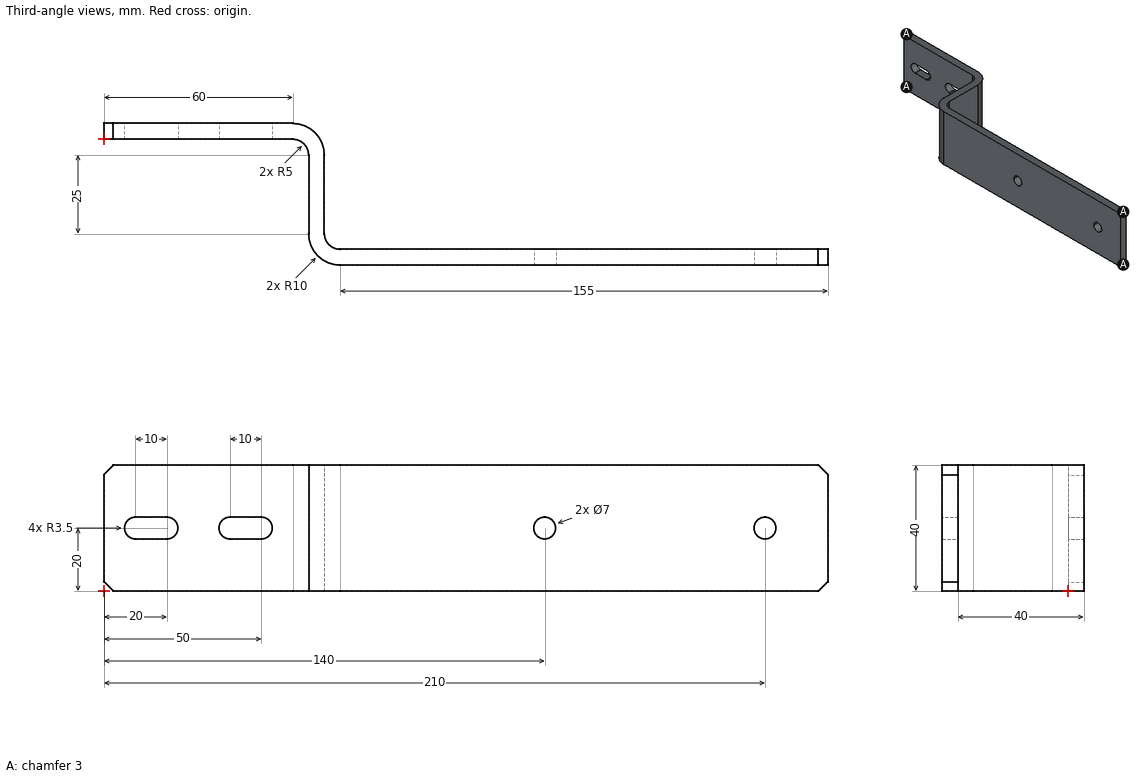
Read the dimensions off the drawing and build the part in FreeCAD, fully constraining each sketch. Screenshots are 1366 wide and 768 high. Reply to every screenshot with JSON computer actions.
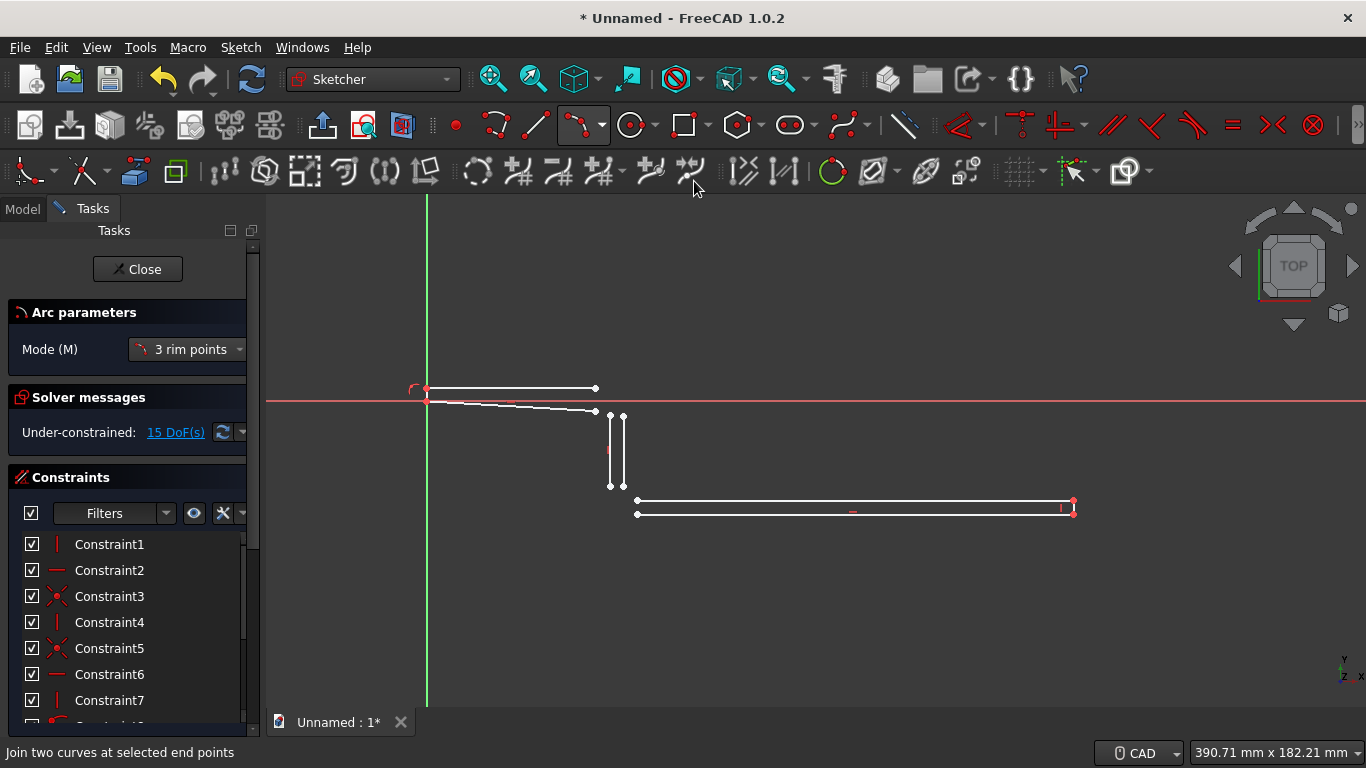
{"action": "left_click", "coordinate": [610, 487]}
{"action": "left_click", "coordinate": [638, 515]}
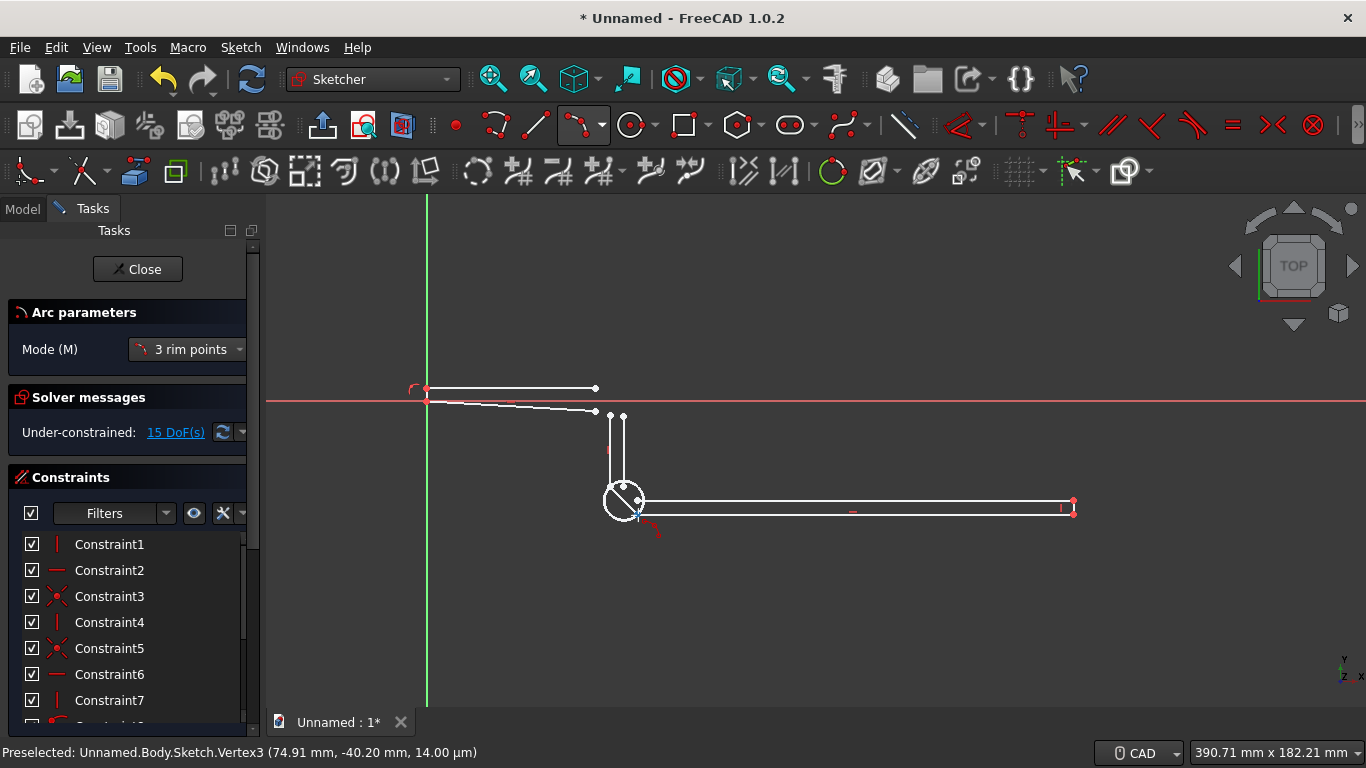
{"action": "scroll", "coordinate": [618, 506], "scroll_direction": "up", "scroll_amount": 4}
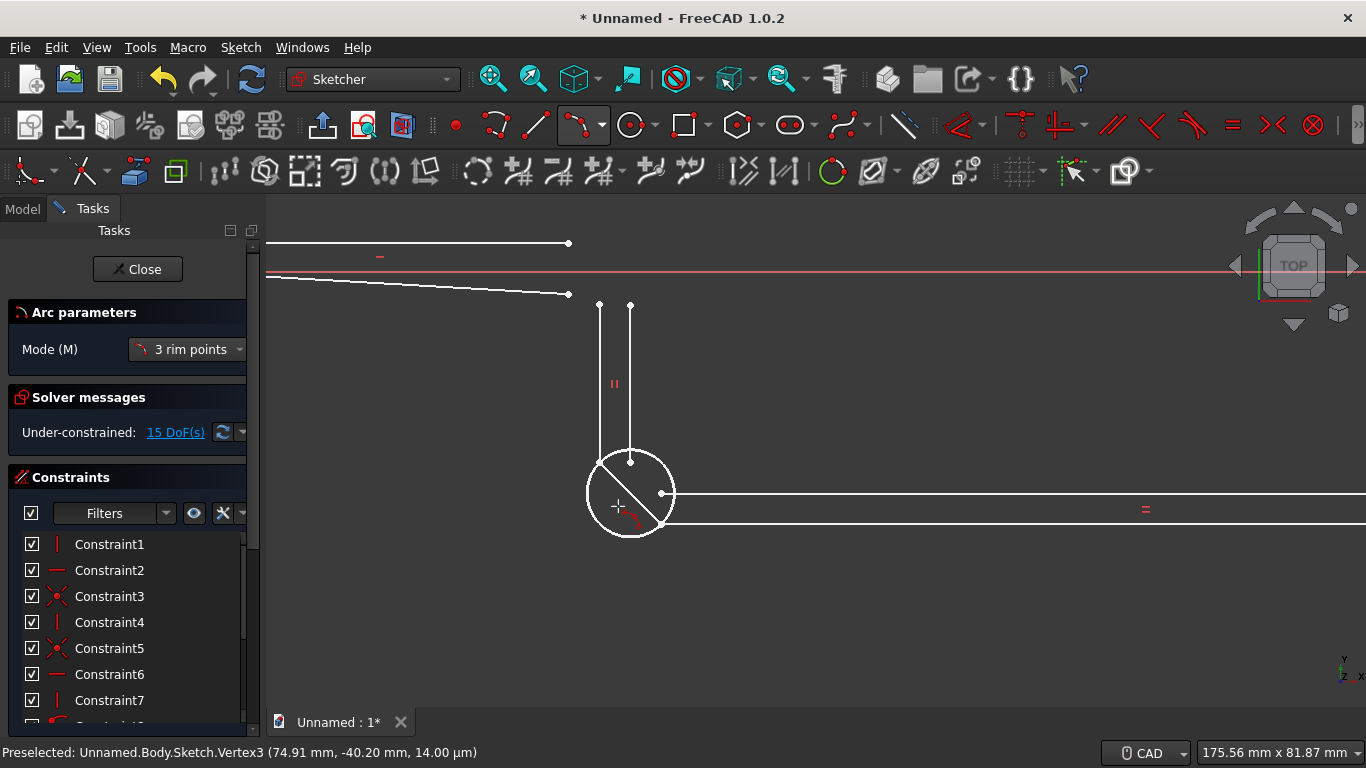
{"action": "left_click", "coordinate": [618, 505]}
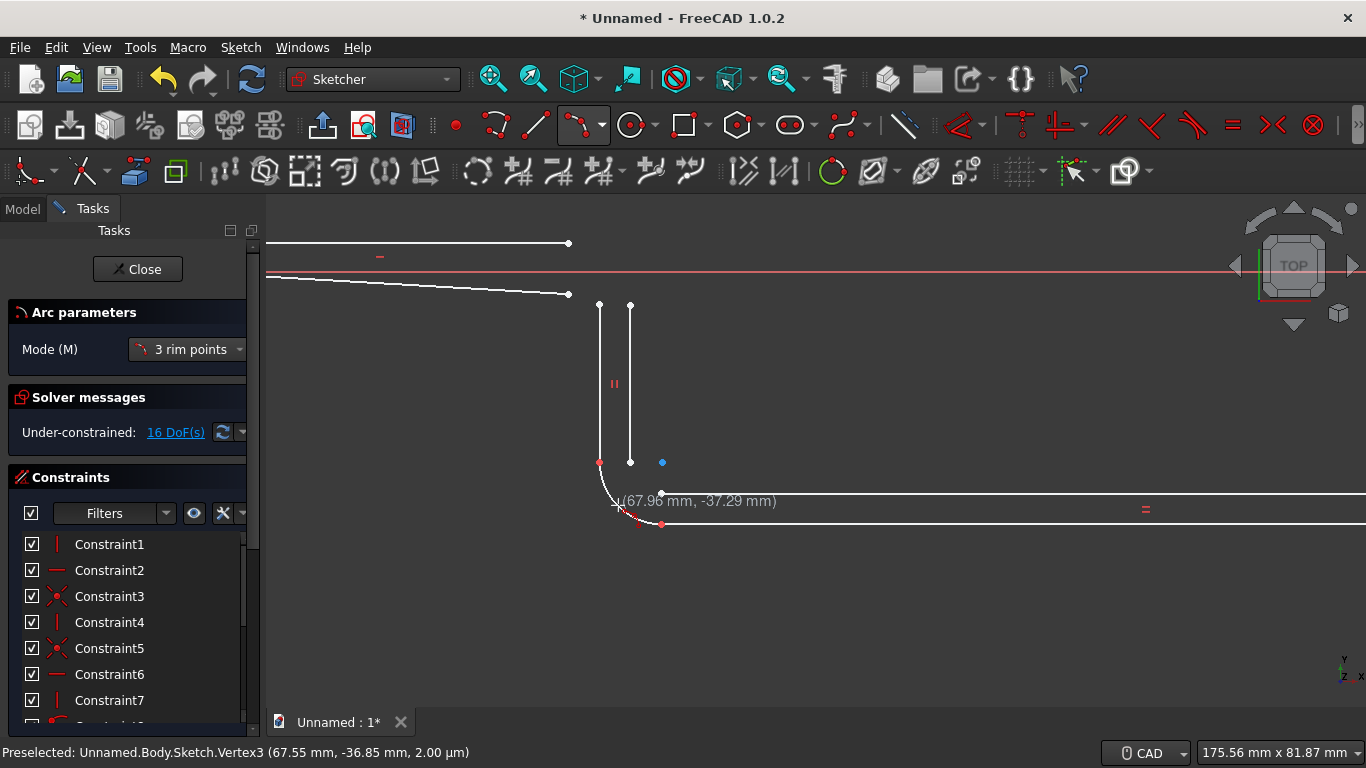
{"action": "left_click", "coordinate": [661, 494]}
{"action": "left_click", "coordinate": [630, 463]}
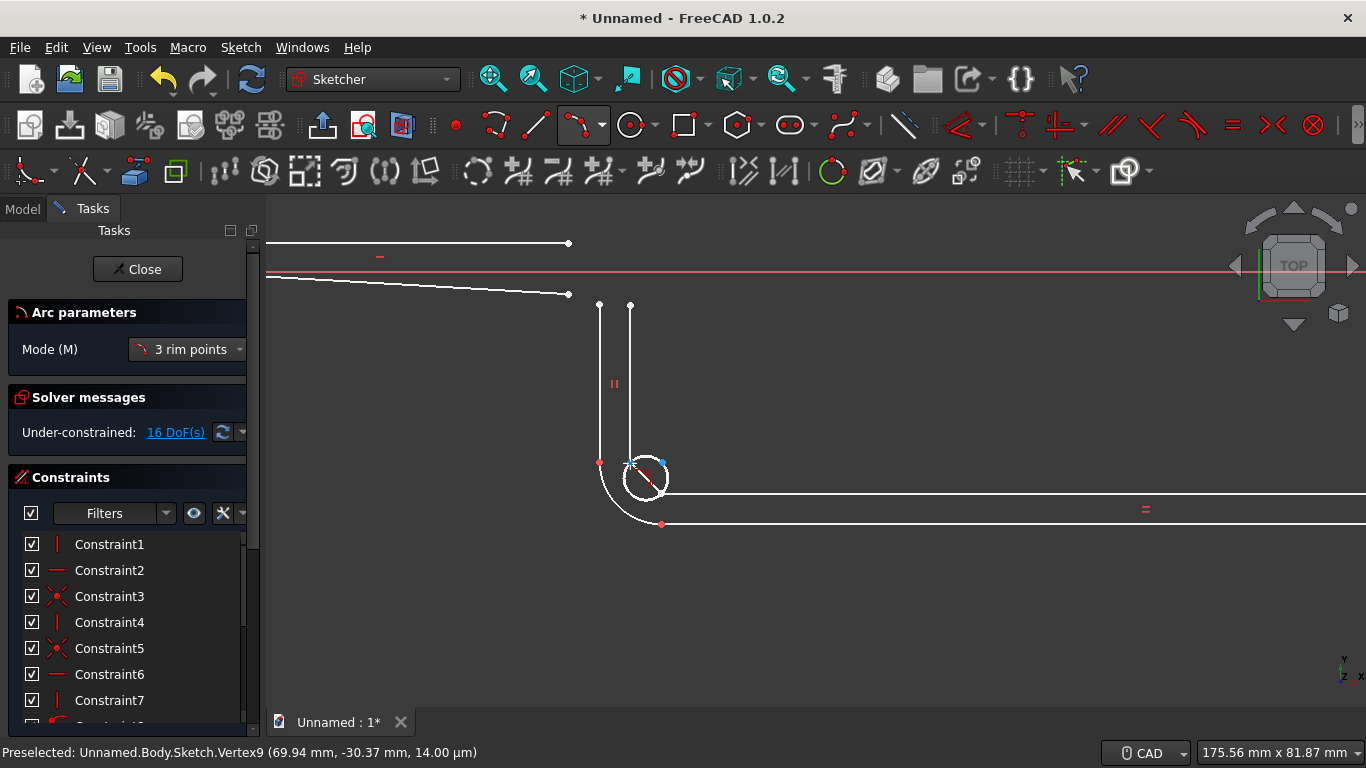
{"action": "scroll", "coordinate": [640, 482], "scroll_direction": "up", "scroll_amount": 3}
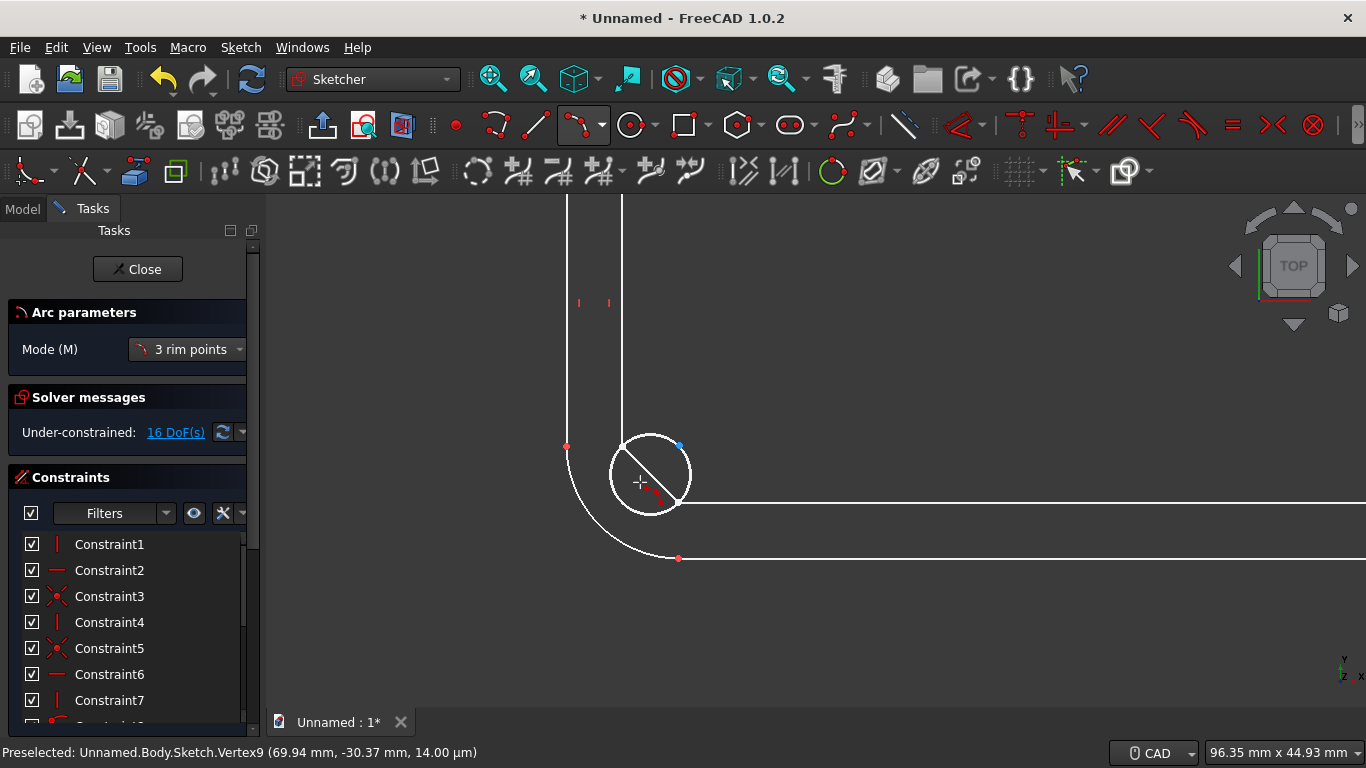
{"action": "left_click", "coordinate": [640, 482]}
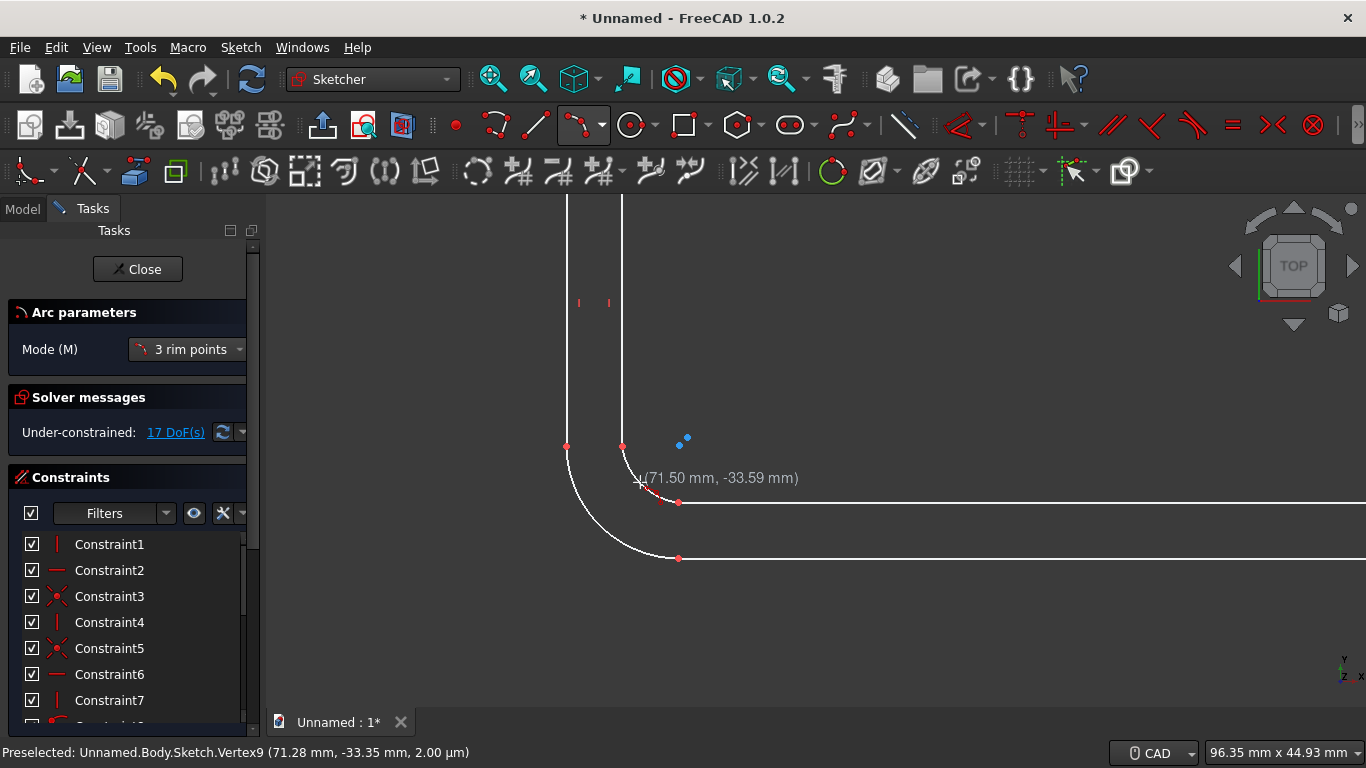
{"action": "scroll", "coordinate": [620, 500], "scroll_direction": "down", "scroll_amount": 7}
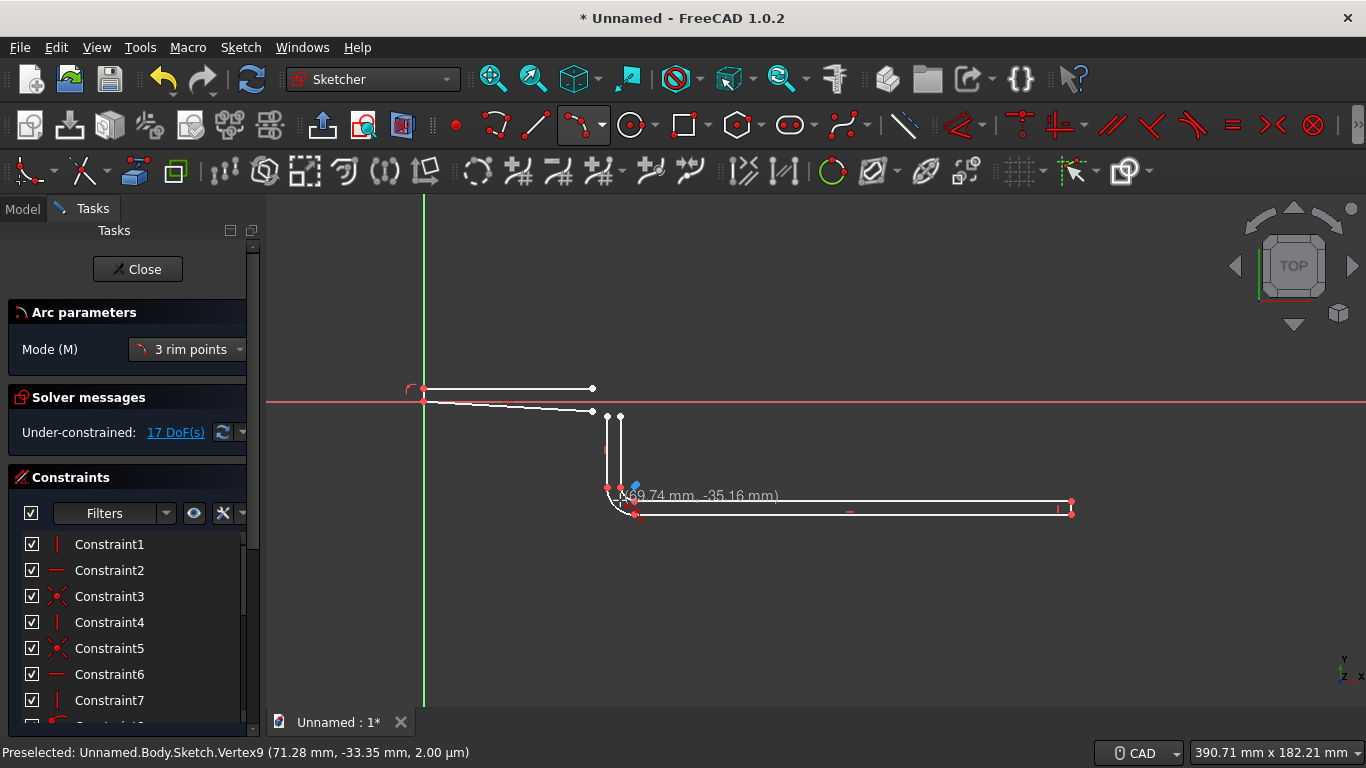
{"action": "left_click", "coordinate": [621, 416]}
{"action": "left_click", "coordinate": [593, 389]}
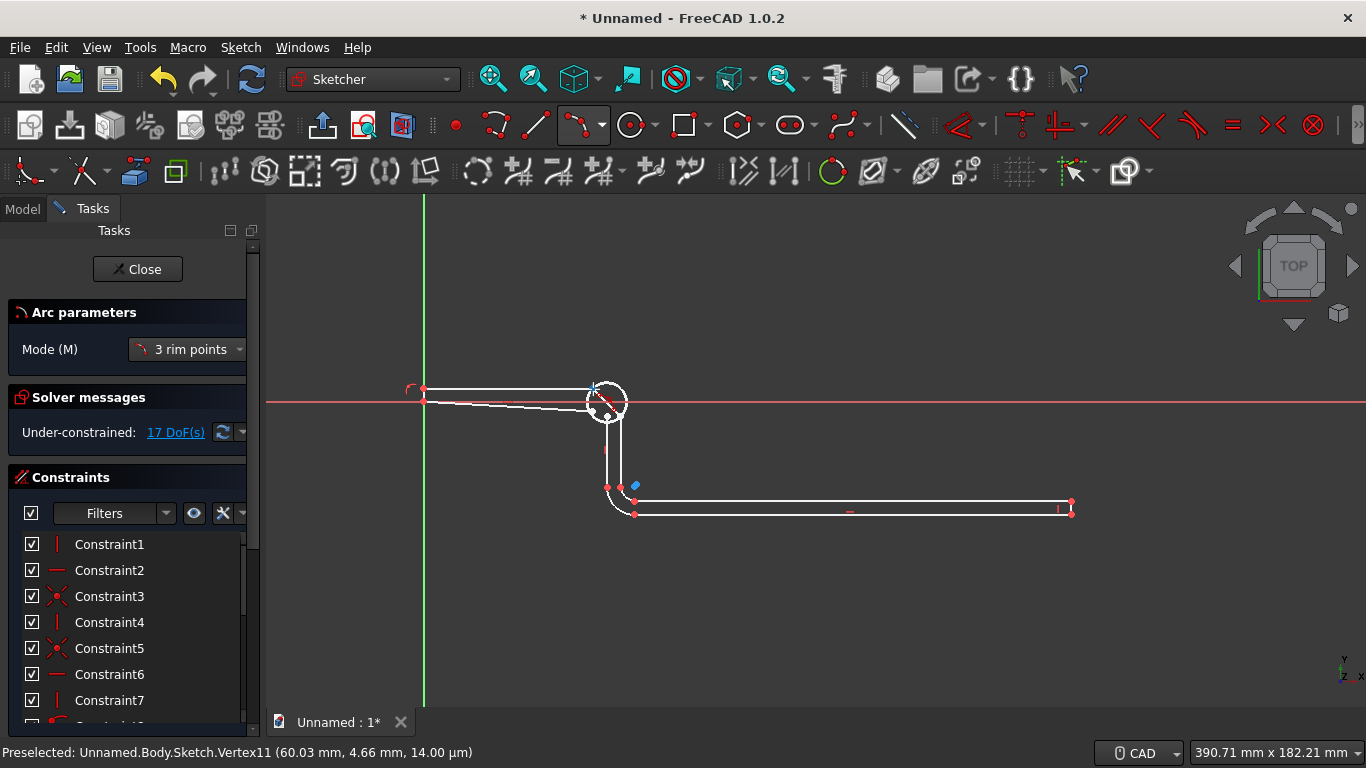
{"action": "scroll", "coordinate": [609, 393], "scroll_direction": "up", "scroll_amount": 4}